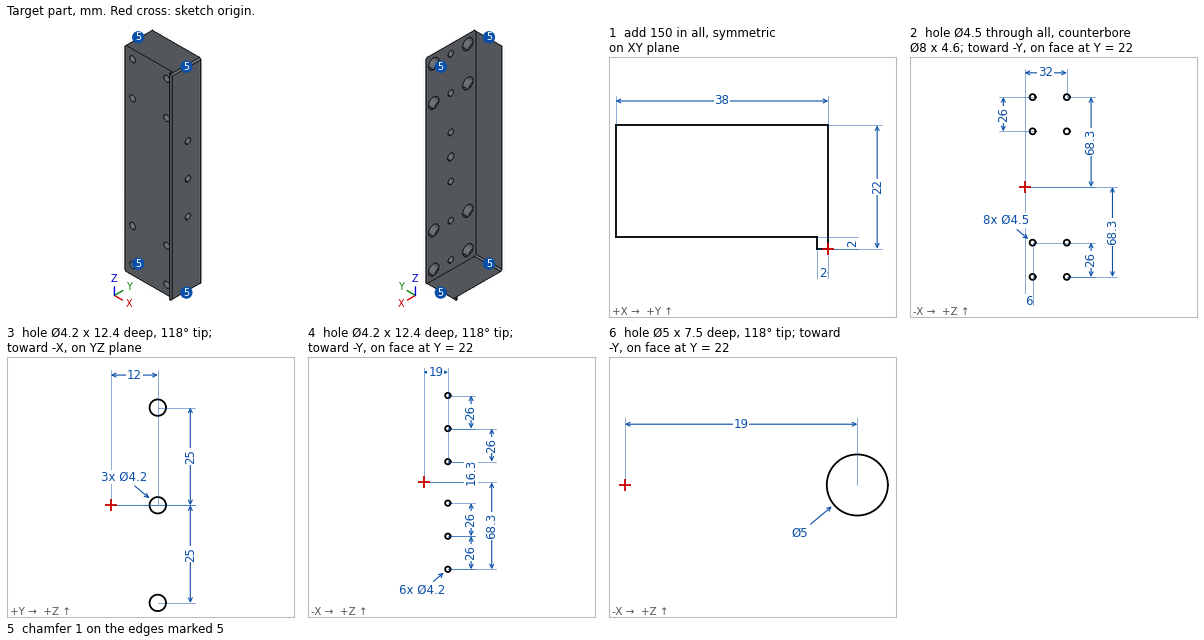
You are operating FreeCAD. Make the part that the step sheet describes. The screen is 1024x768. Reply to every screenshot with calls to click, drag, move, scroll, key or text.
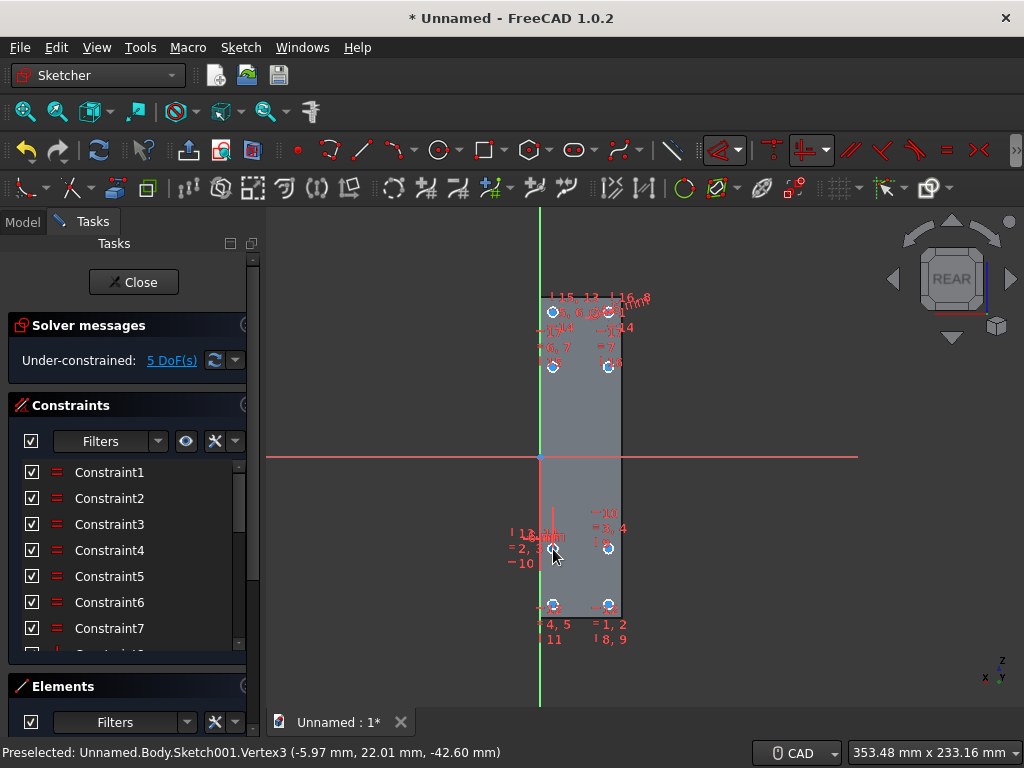
click(609, 312)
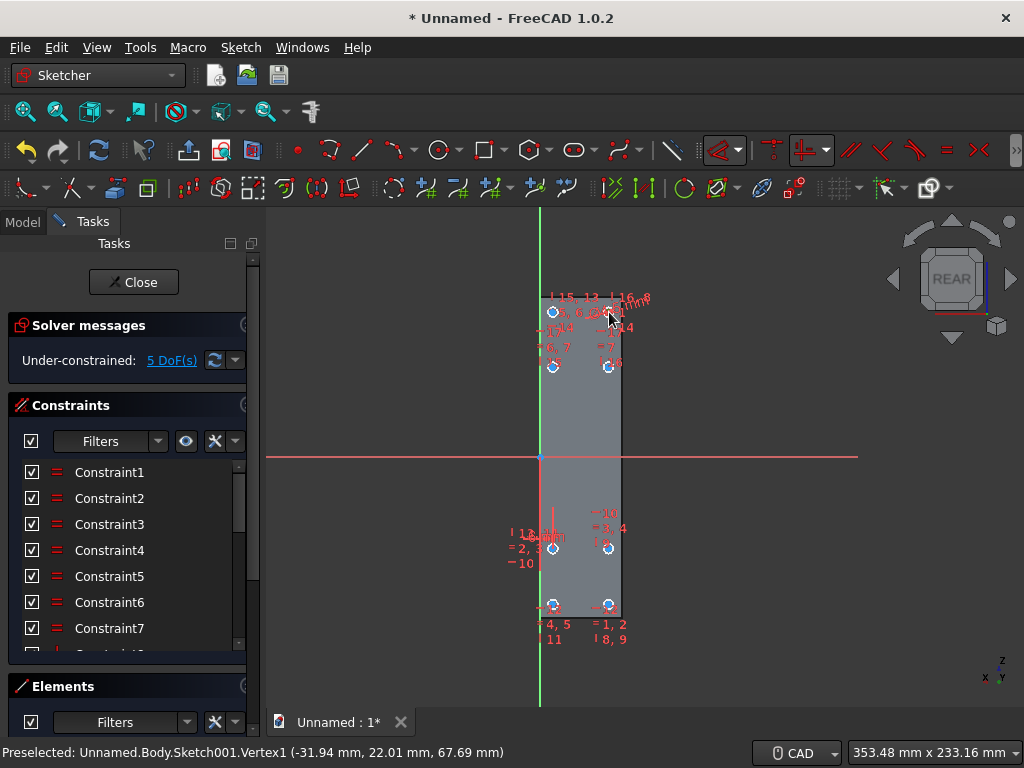
key(l)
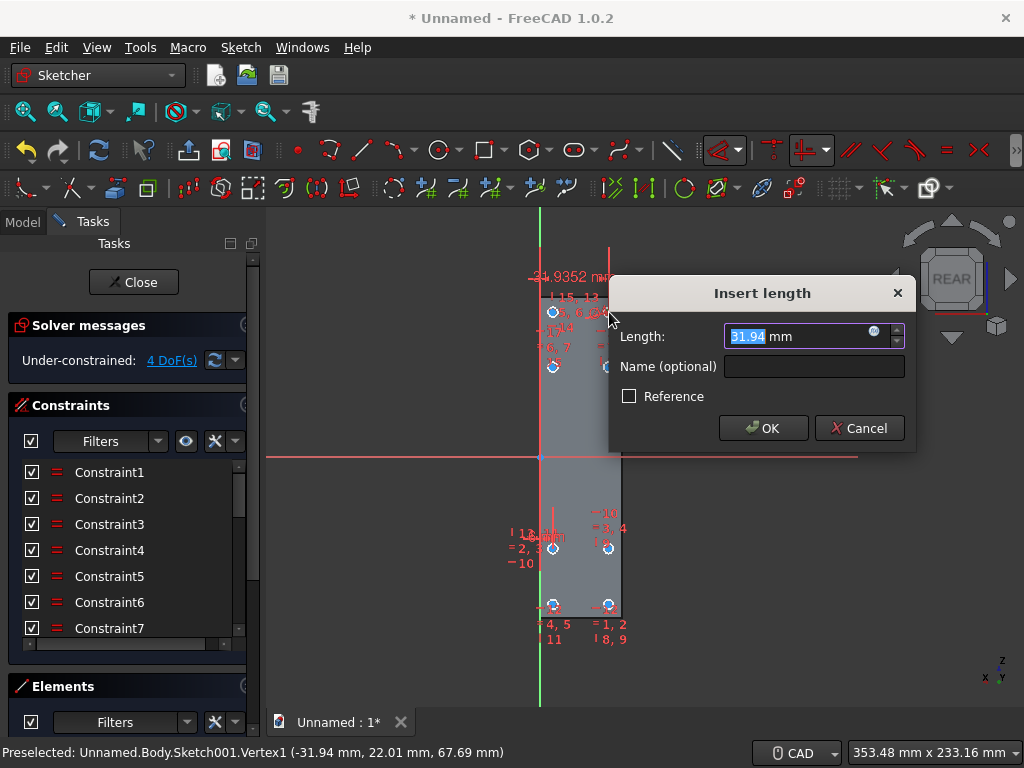
text(32)
key(Return)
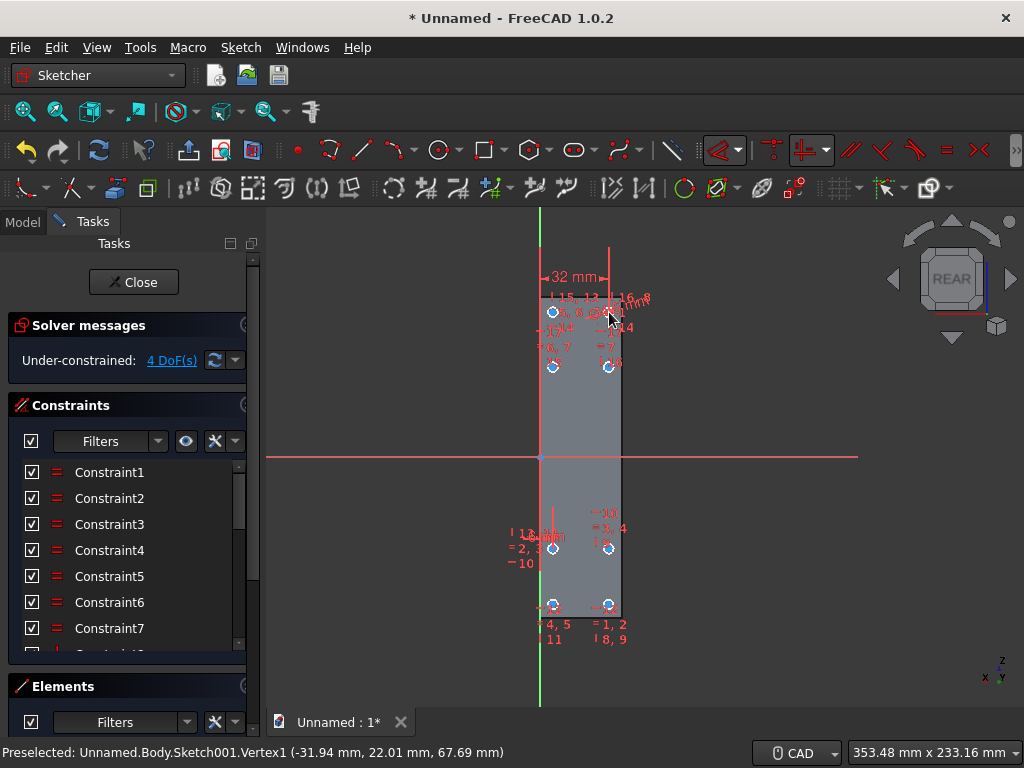
click(609, 604)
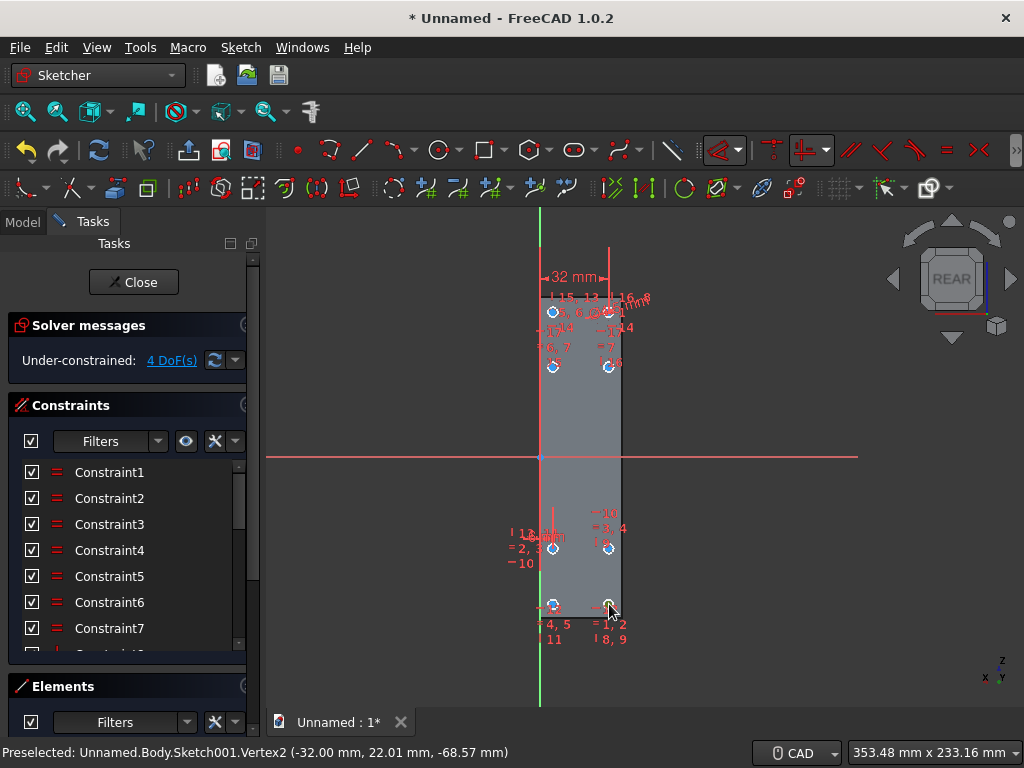
click(553, 549)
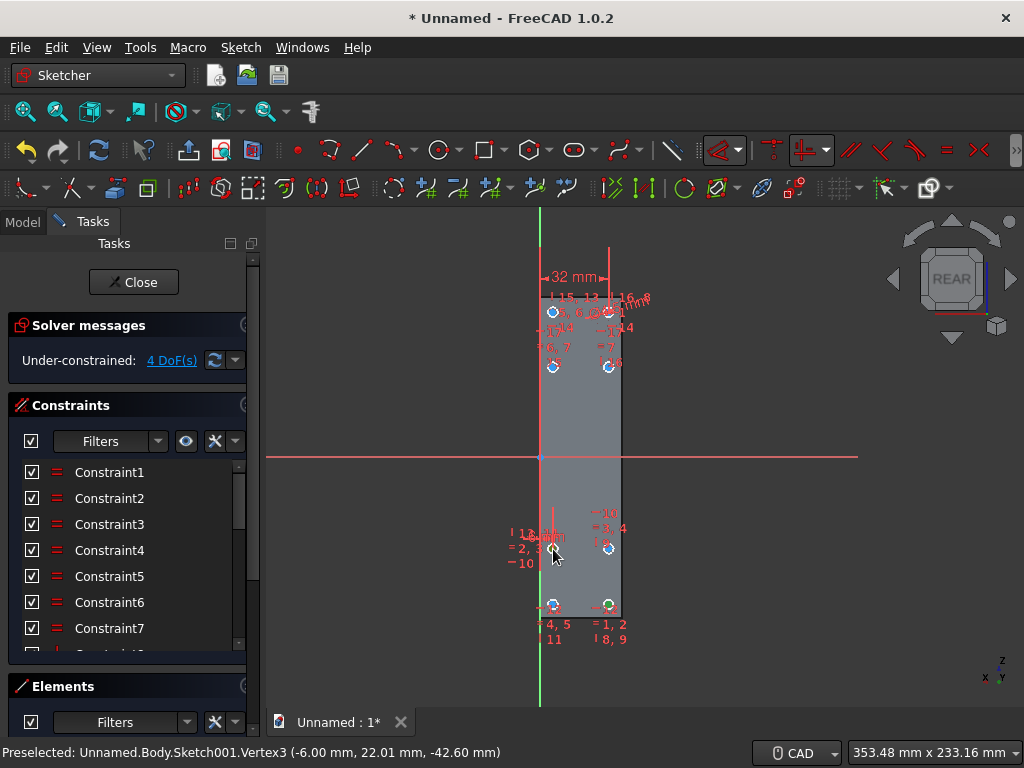
key(i)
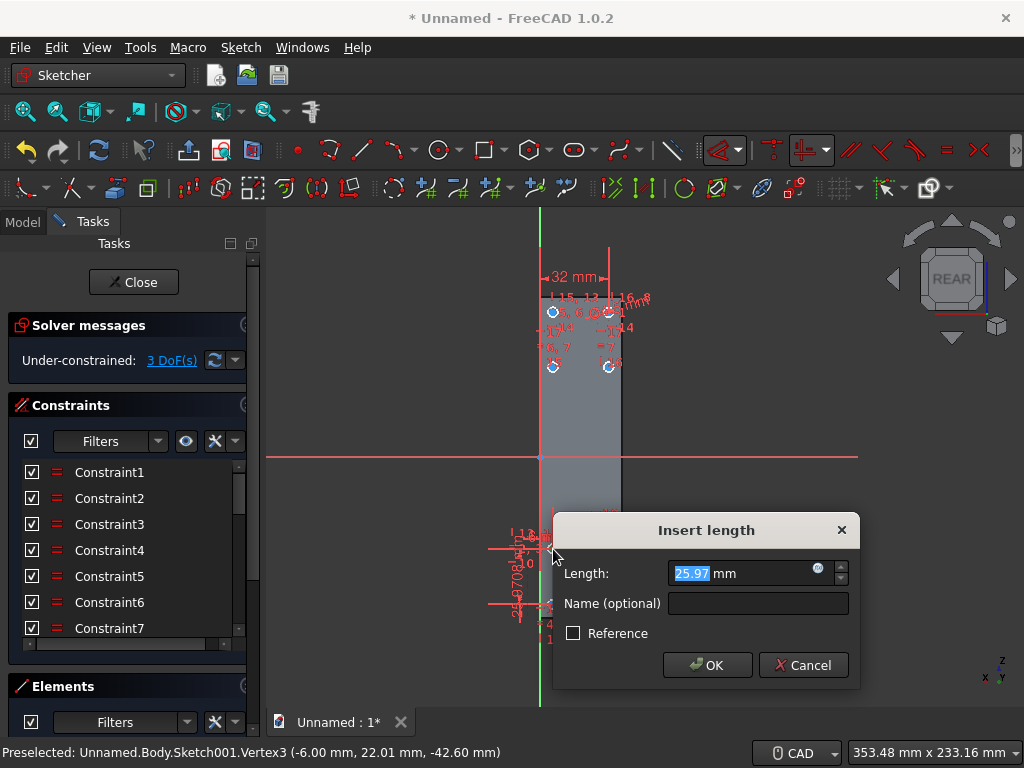
text(26)
key(Return)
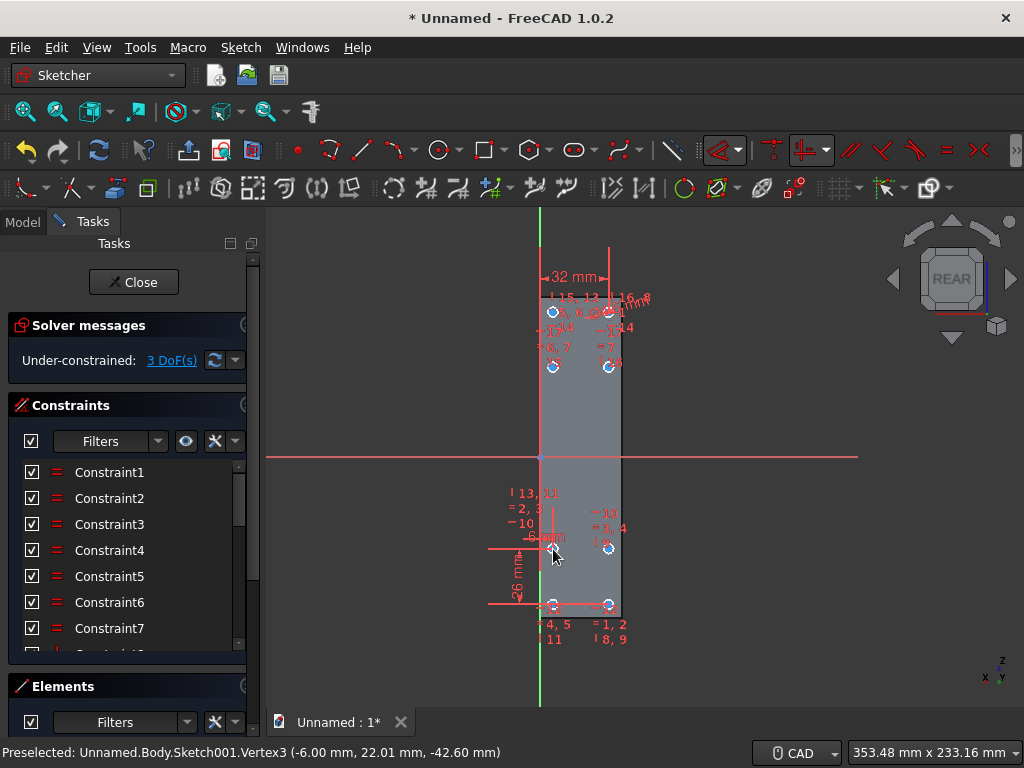
click(553, 312)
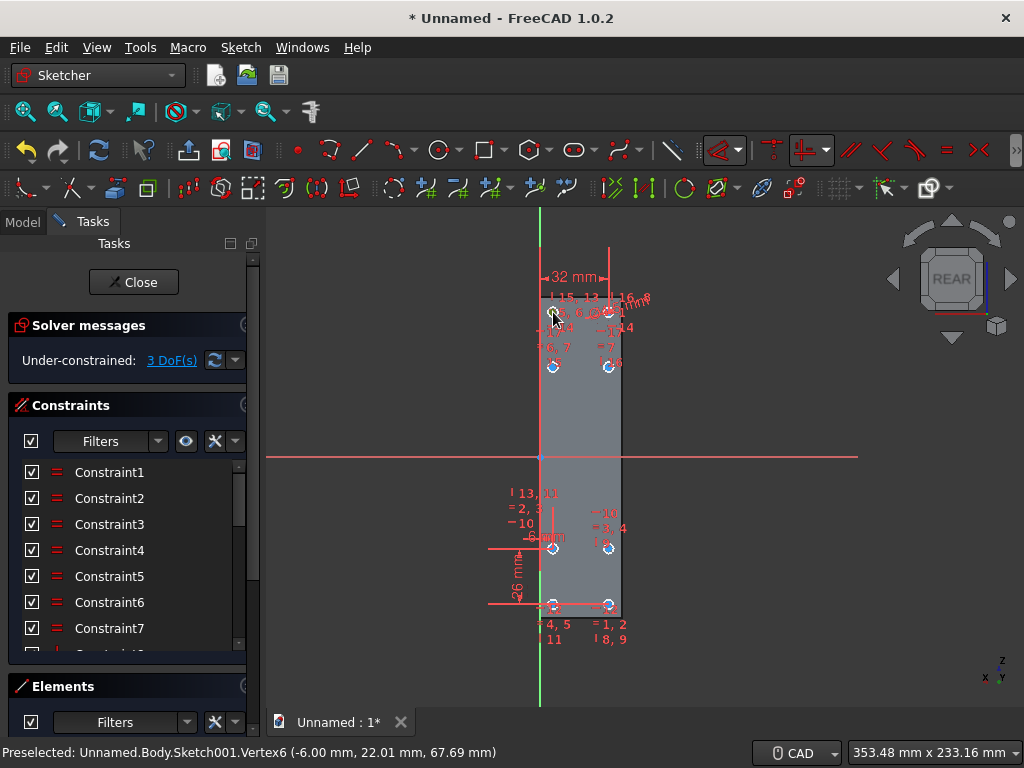
click(553, 367)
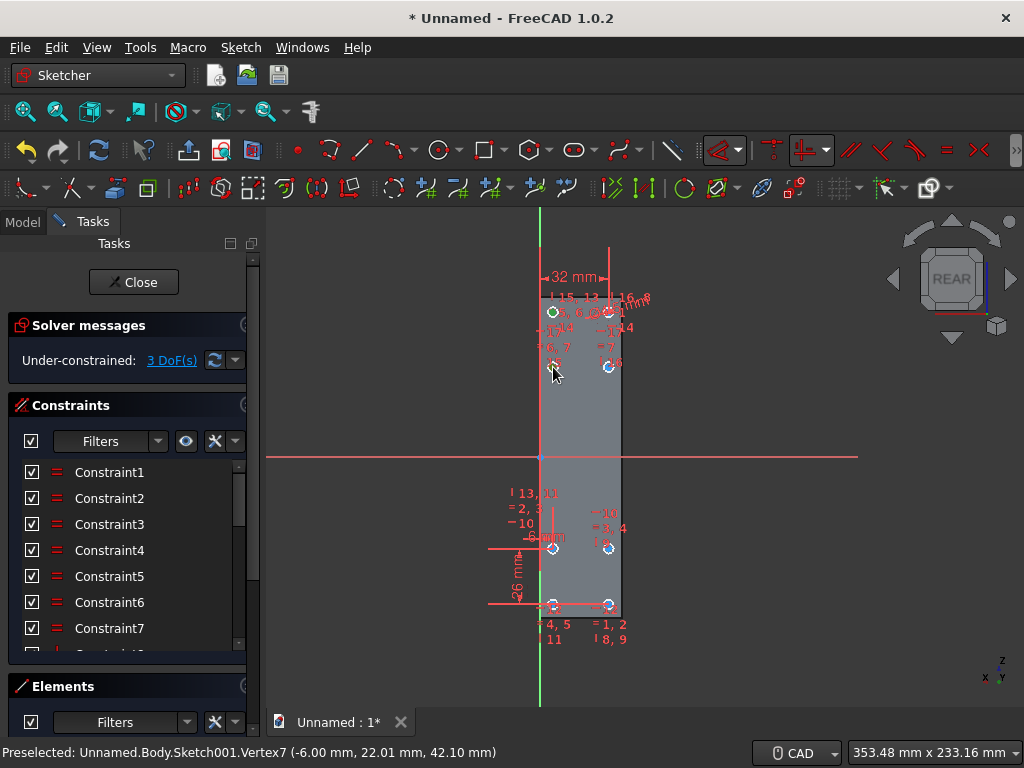
key(i)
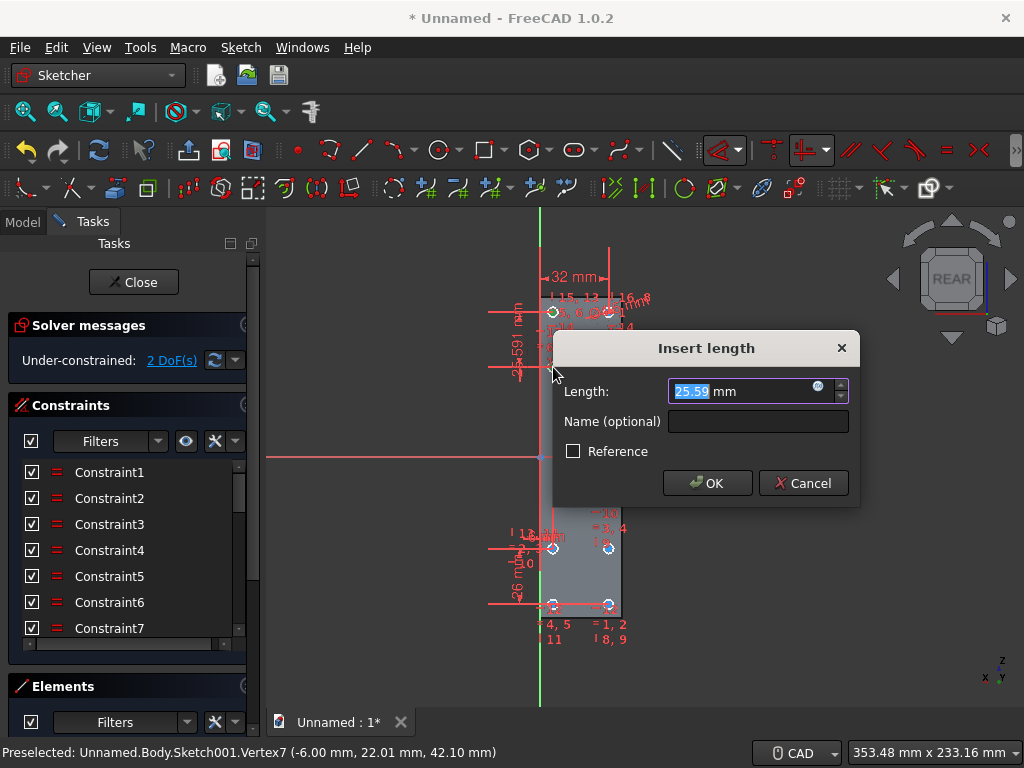
text(26)
key(Return)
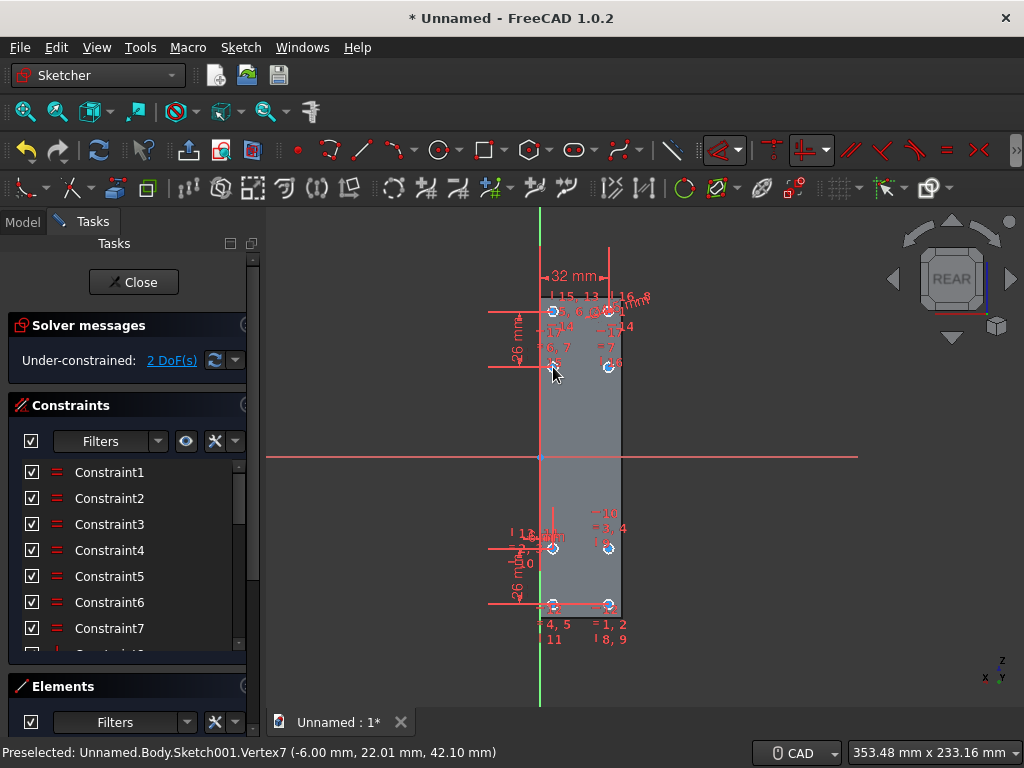
click(609, 312)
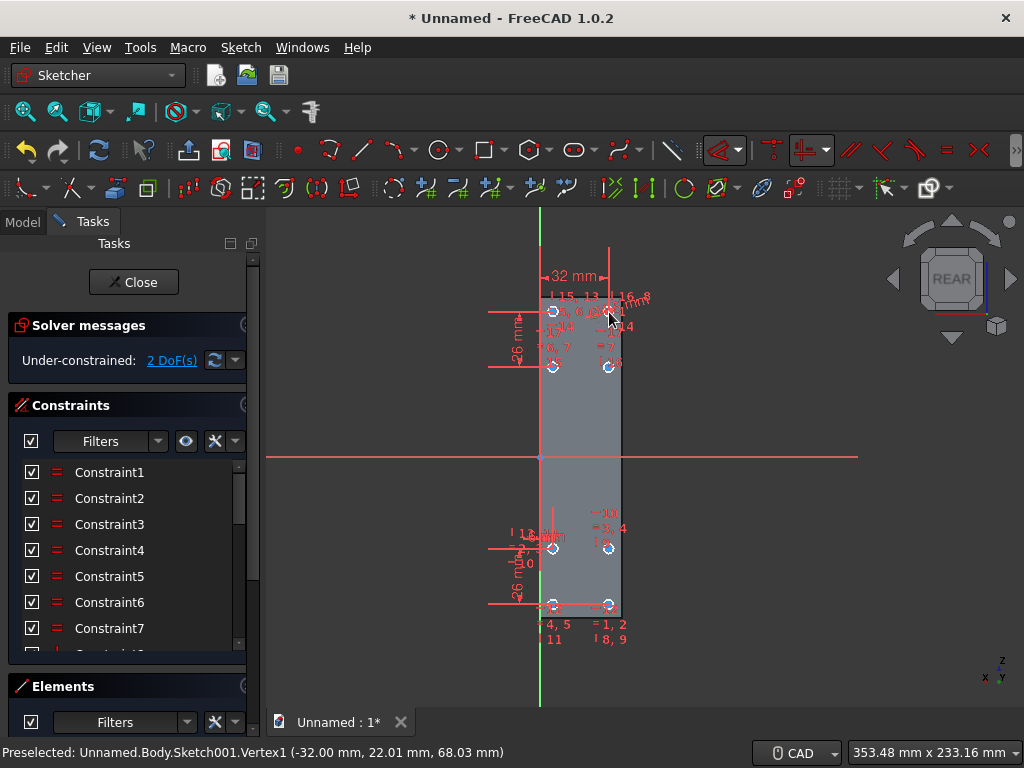
key(i)